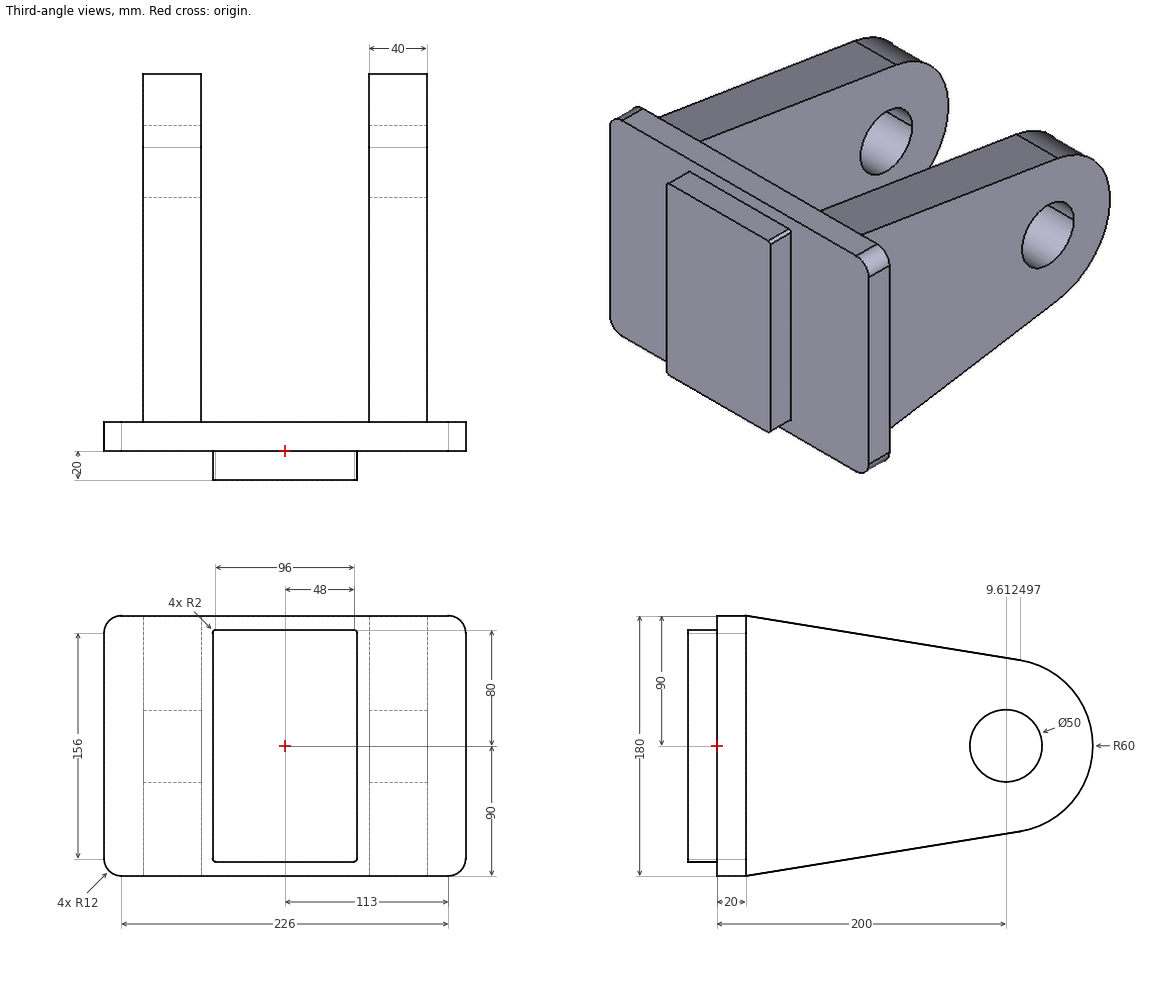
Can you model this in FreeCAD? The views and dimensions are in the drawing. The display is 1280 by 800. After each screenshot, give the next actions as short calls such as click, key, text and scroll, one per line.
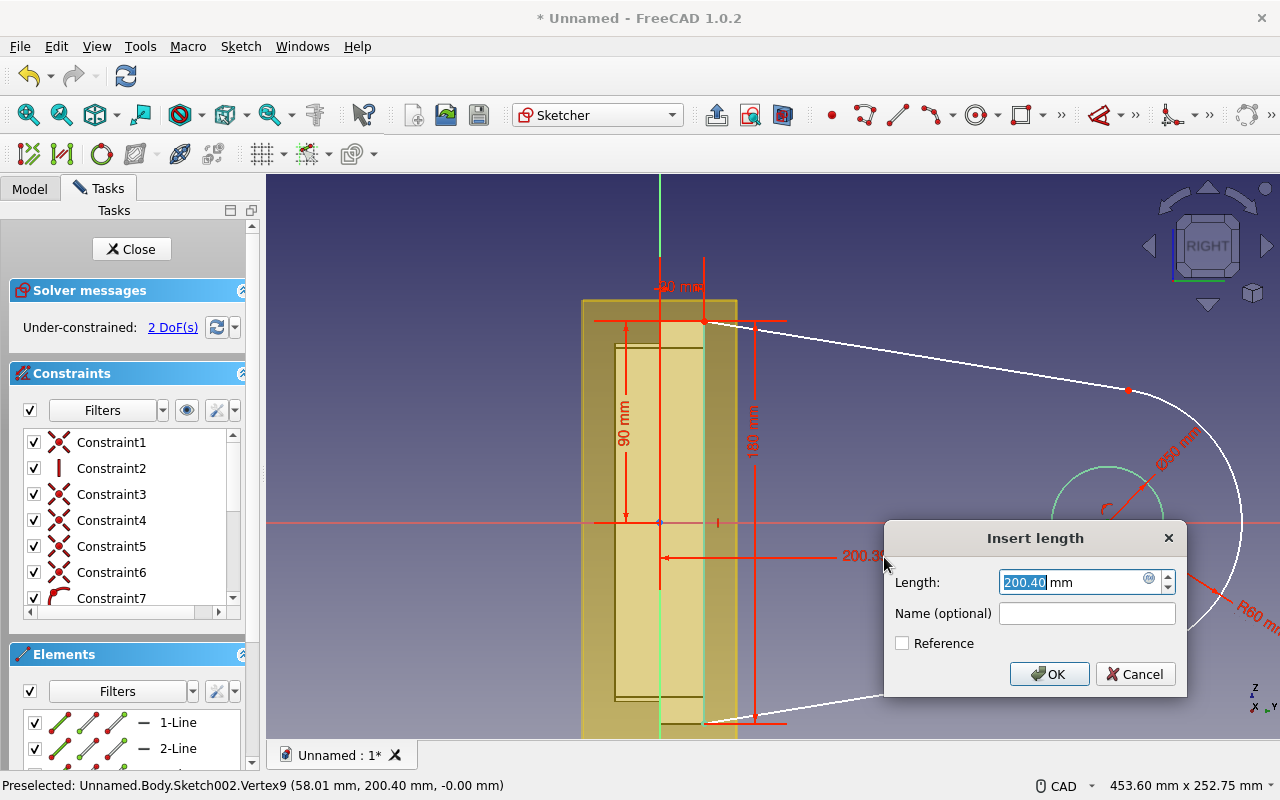
text(200)
key(Return)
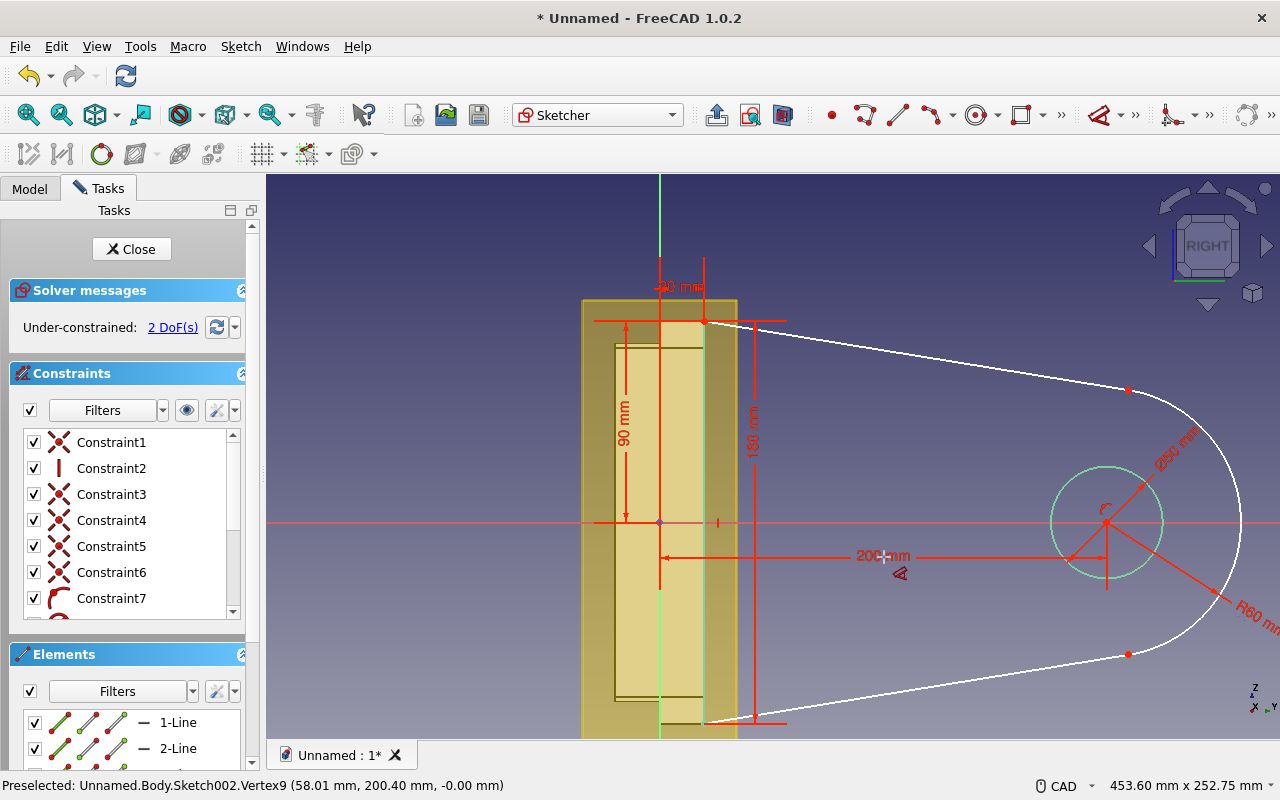
scroll(294, 202, down, 1)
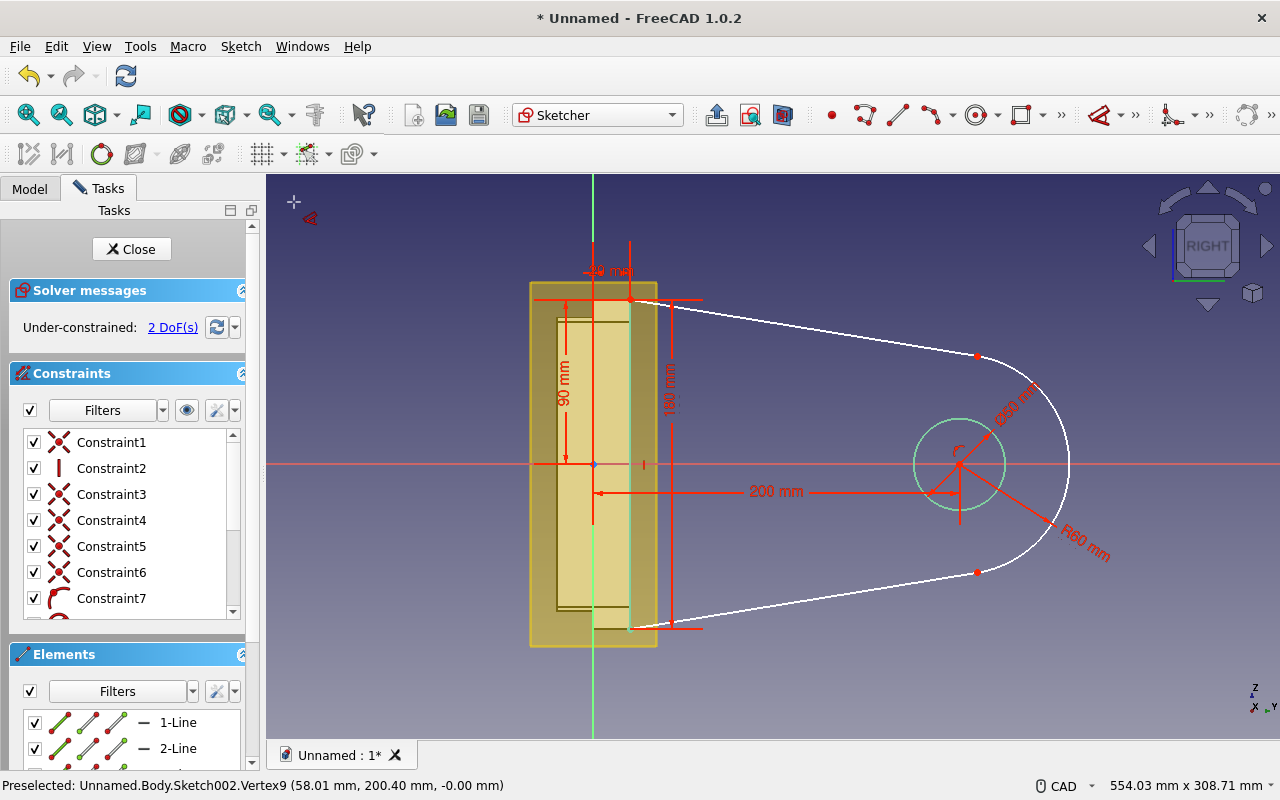
scroll(977, 356, up, 5)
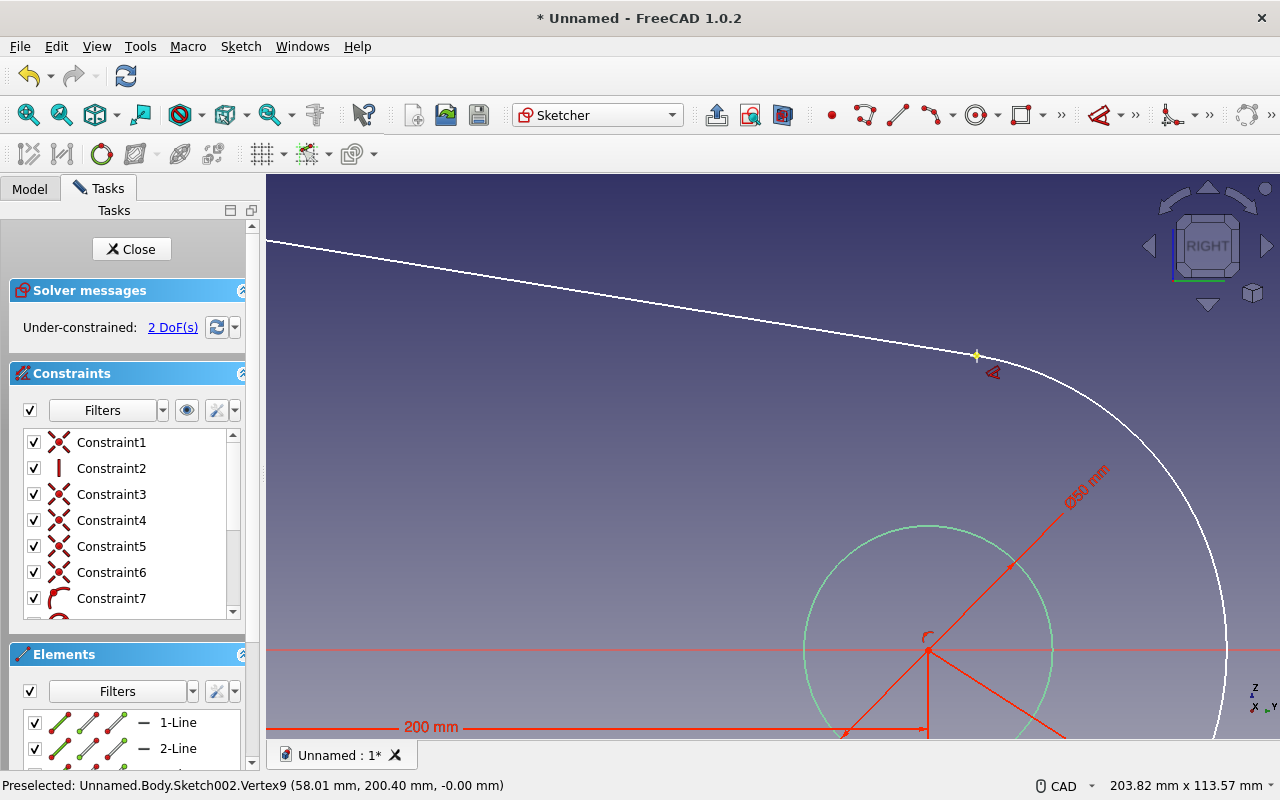
click(976, 356)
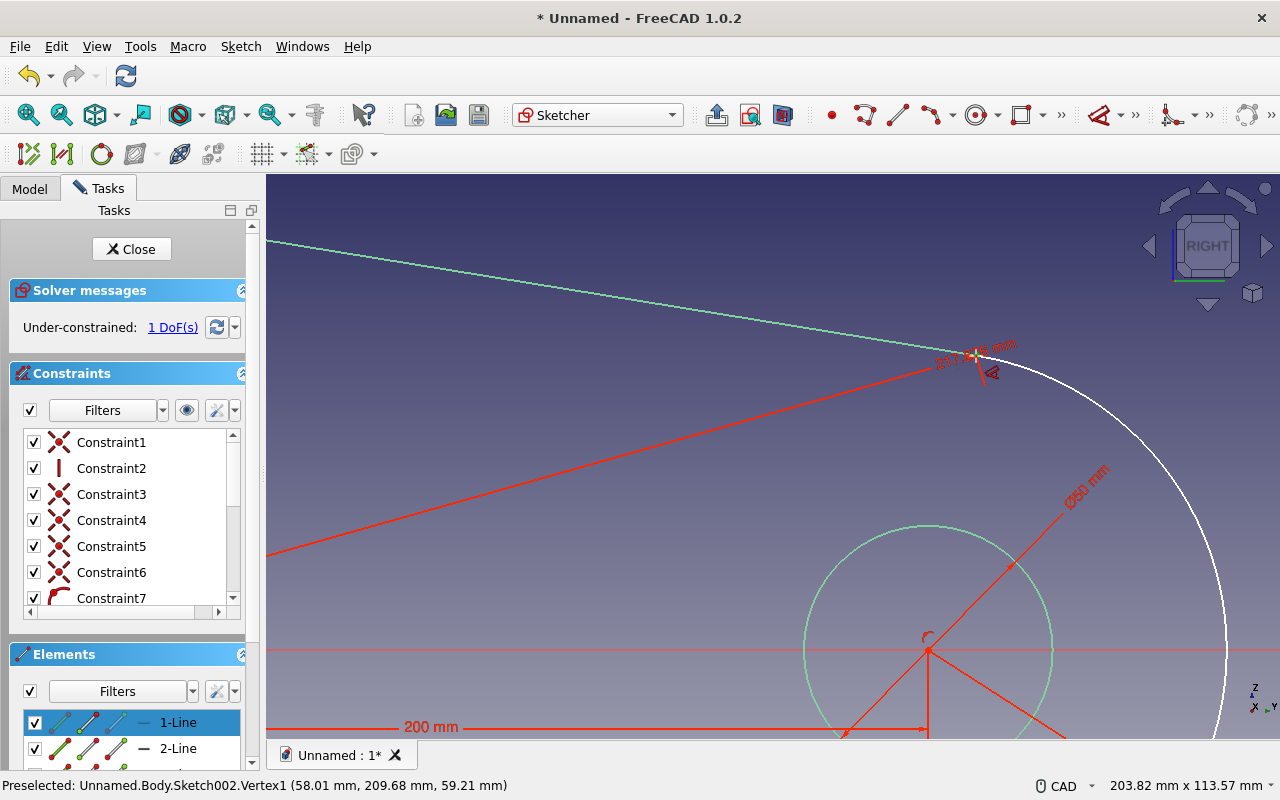
click(928, 650)
click(952, 322)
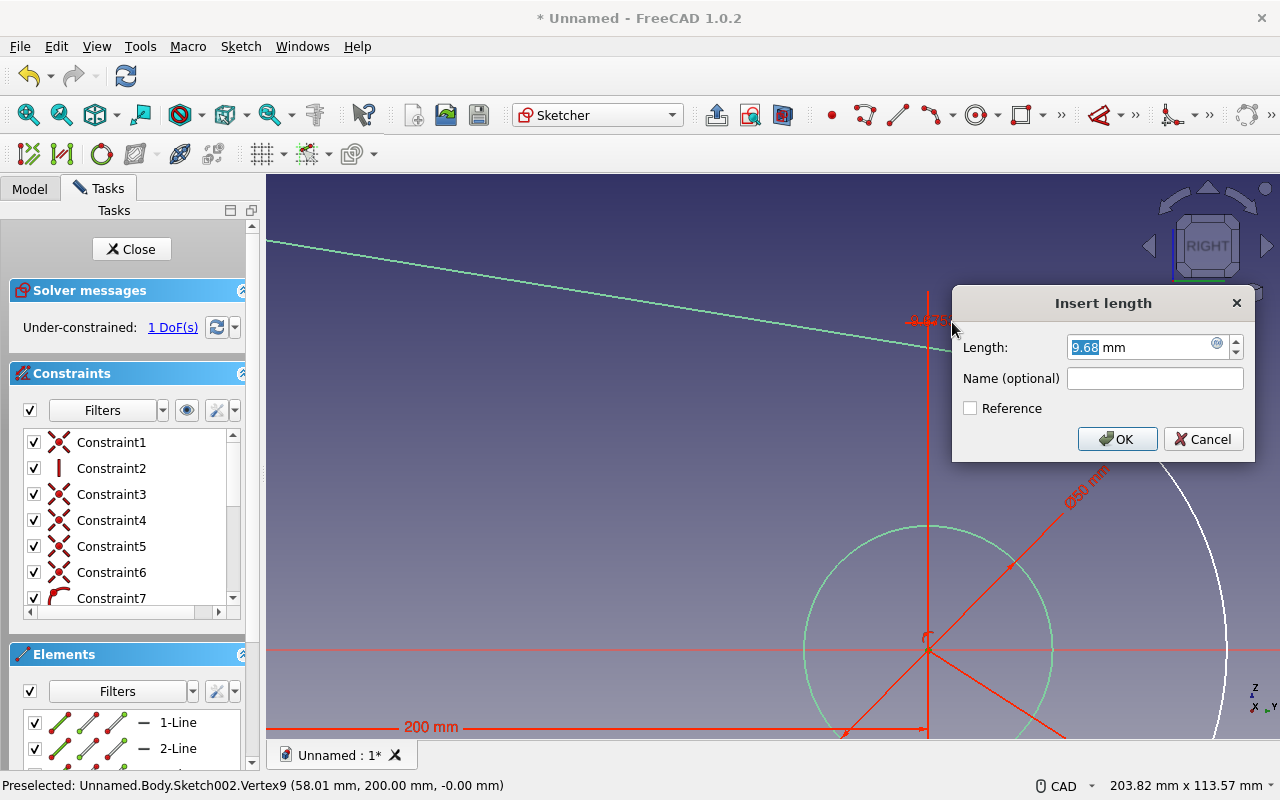
text(9.612497)
key(Return)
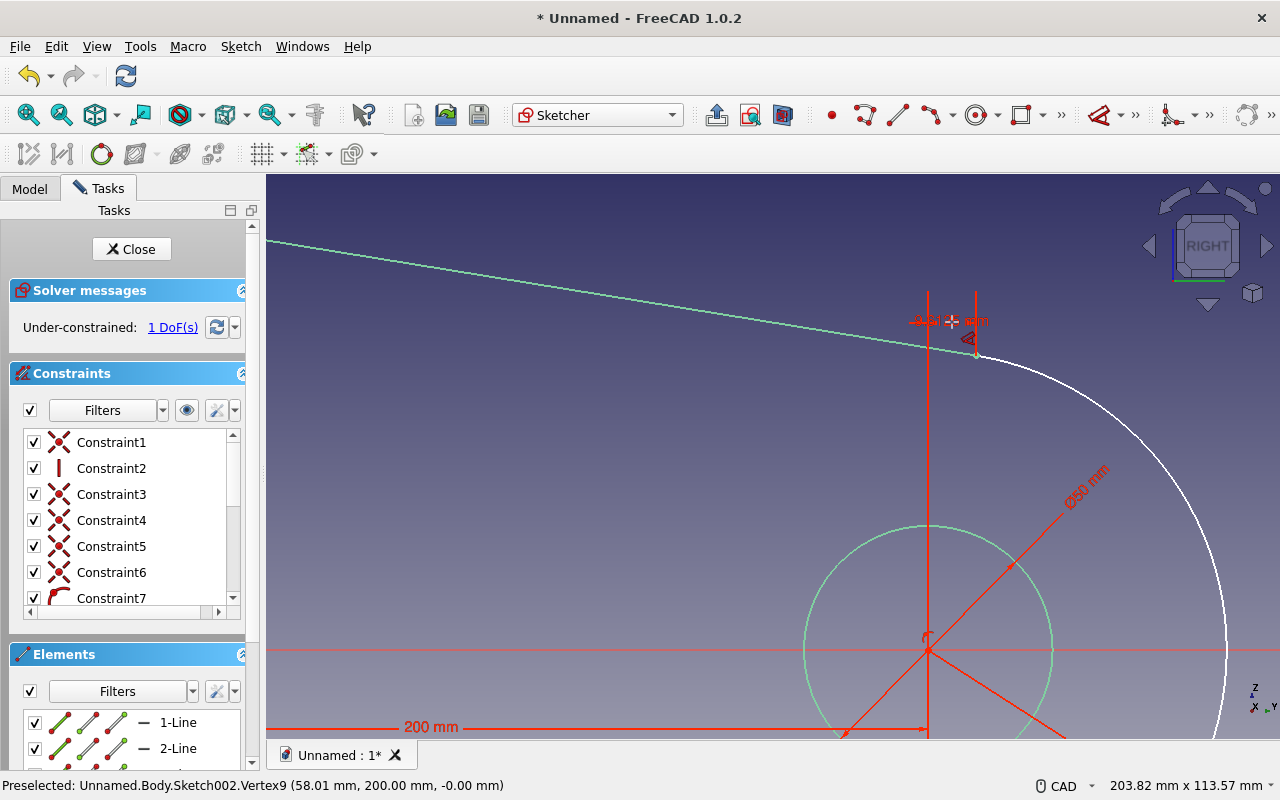
scroll(777, 344, down, 5)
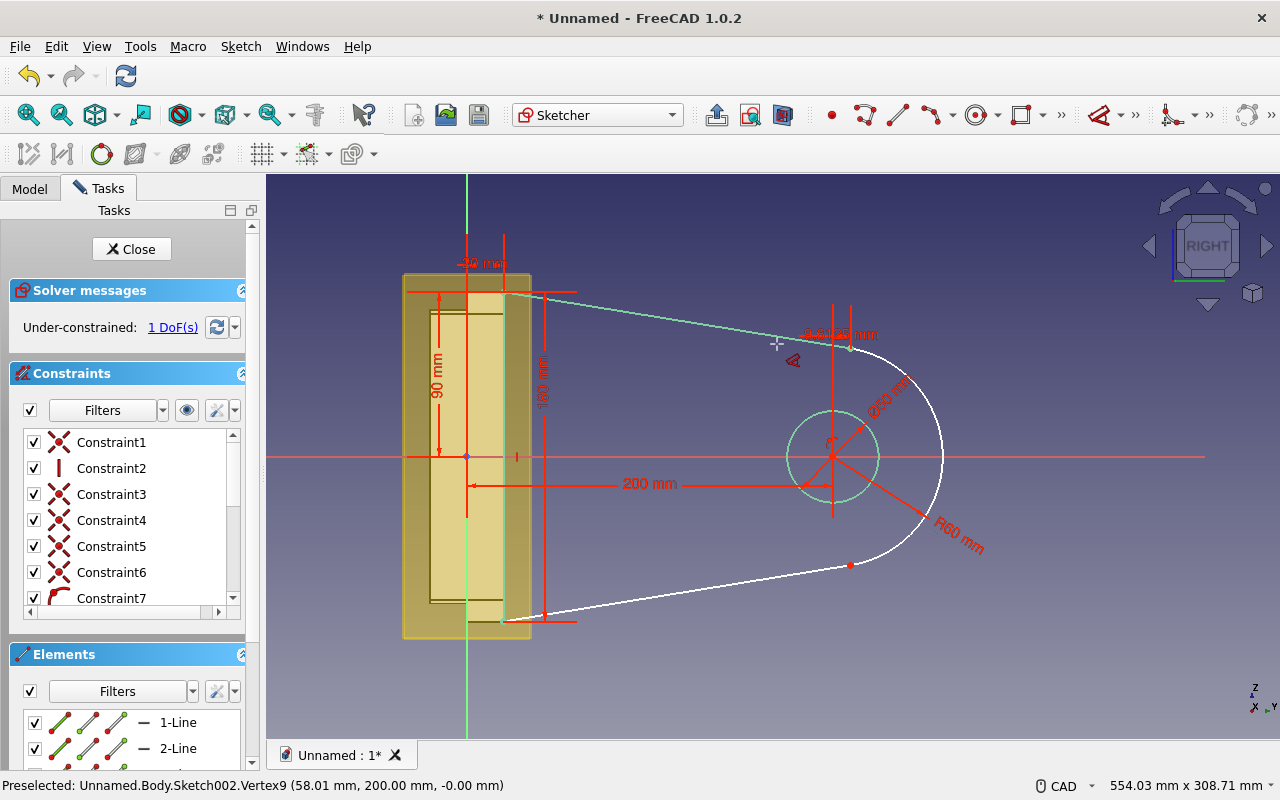
scroll(851, 565, up, 5)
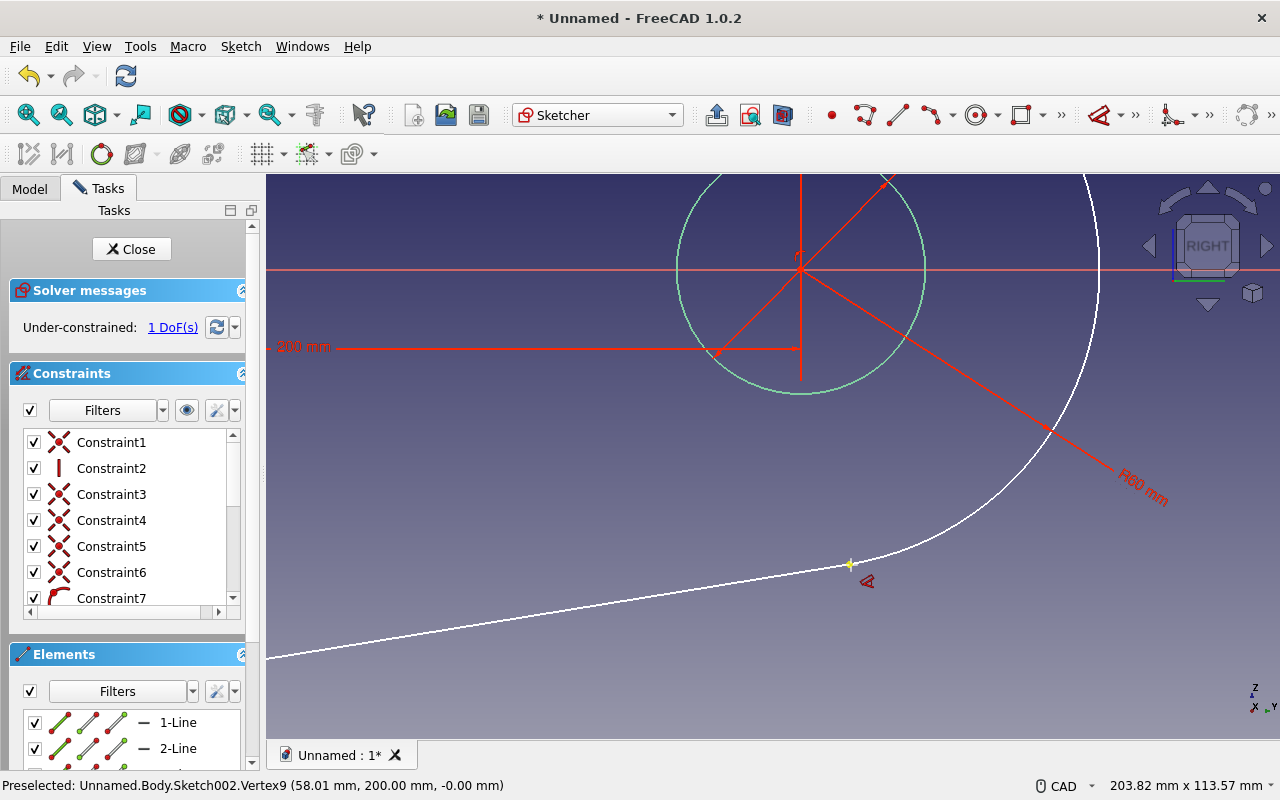
click(849, 564)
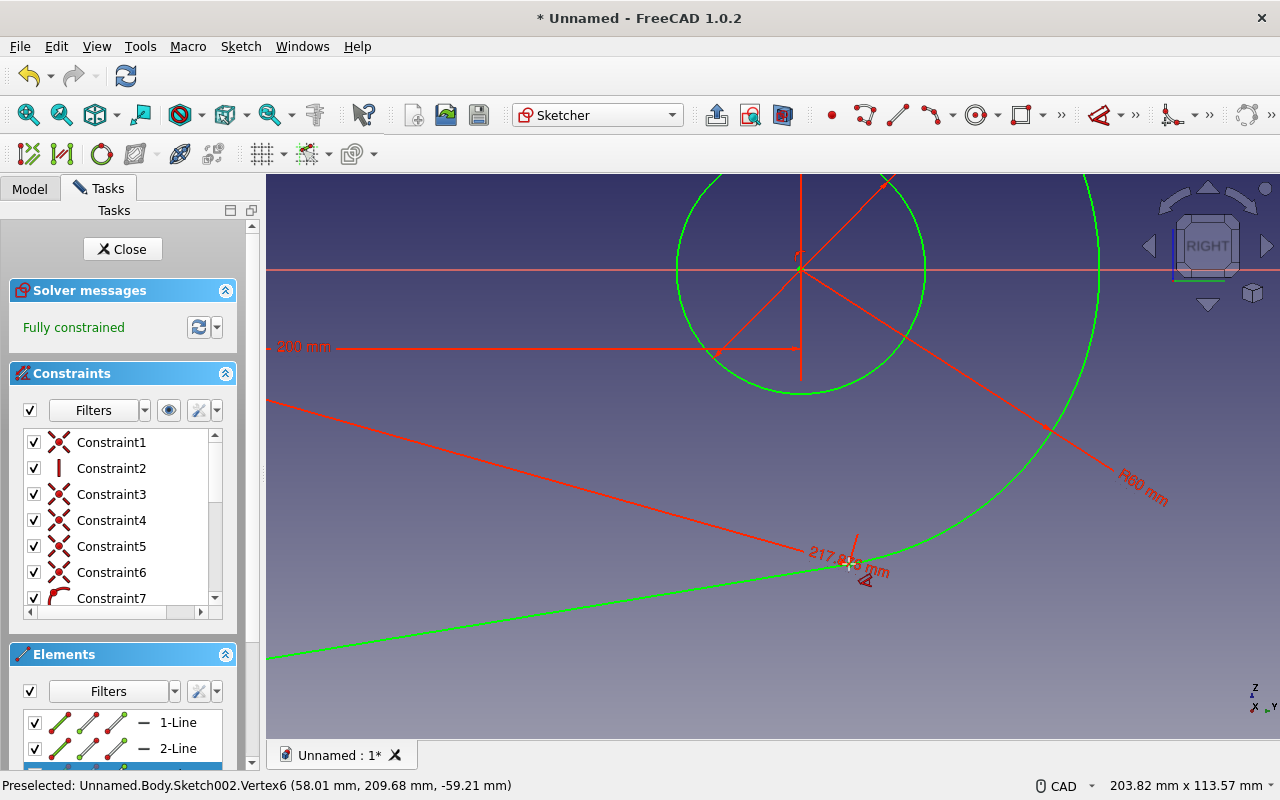
click(801, 270)
click(825, 598)